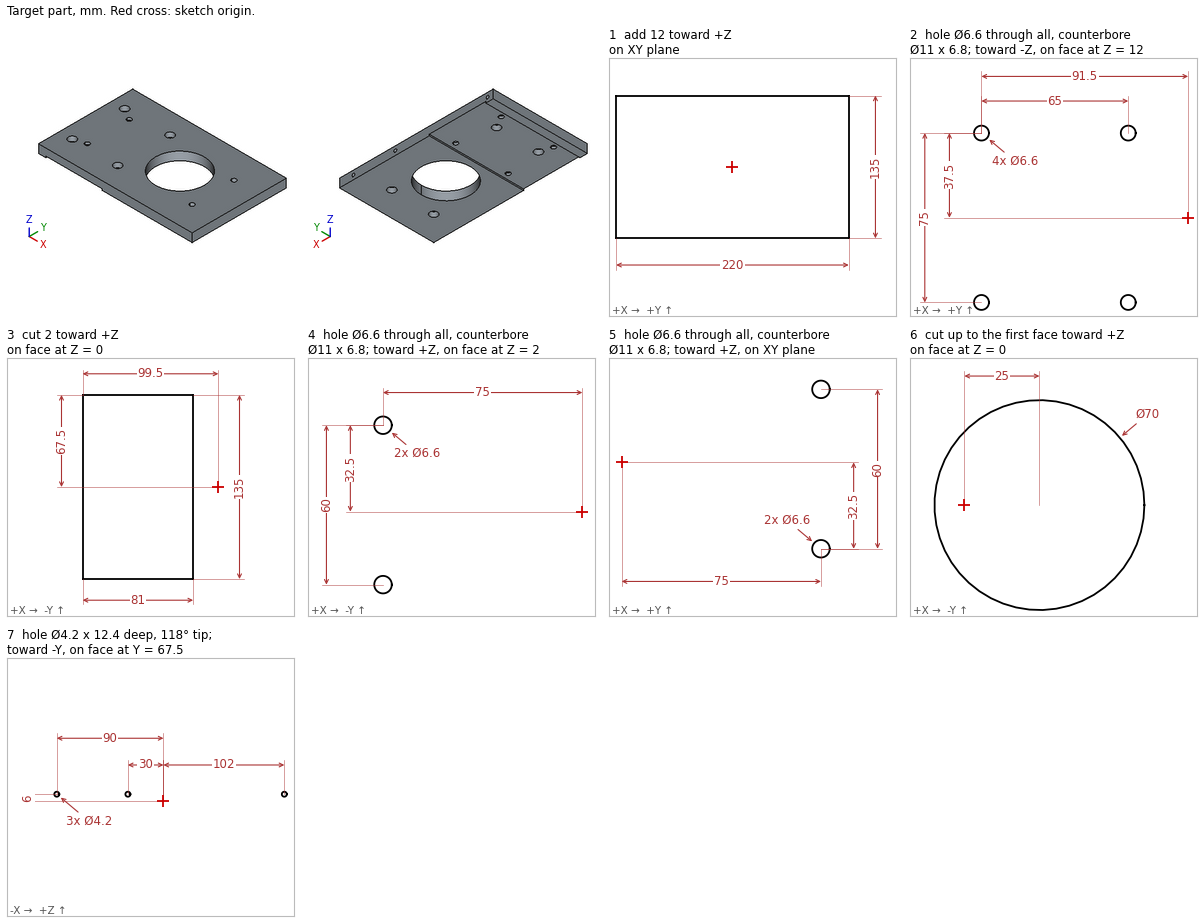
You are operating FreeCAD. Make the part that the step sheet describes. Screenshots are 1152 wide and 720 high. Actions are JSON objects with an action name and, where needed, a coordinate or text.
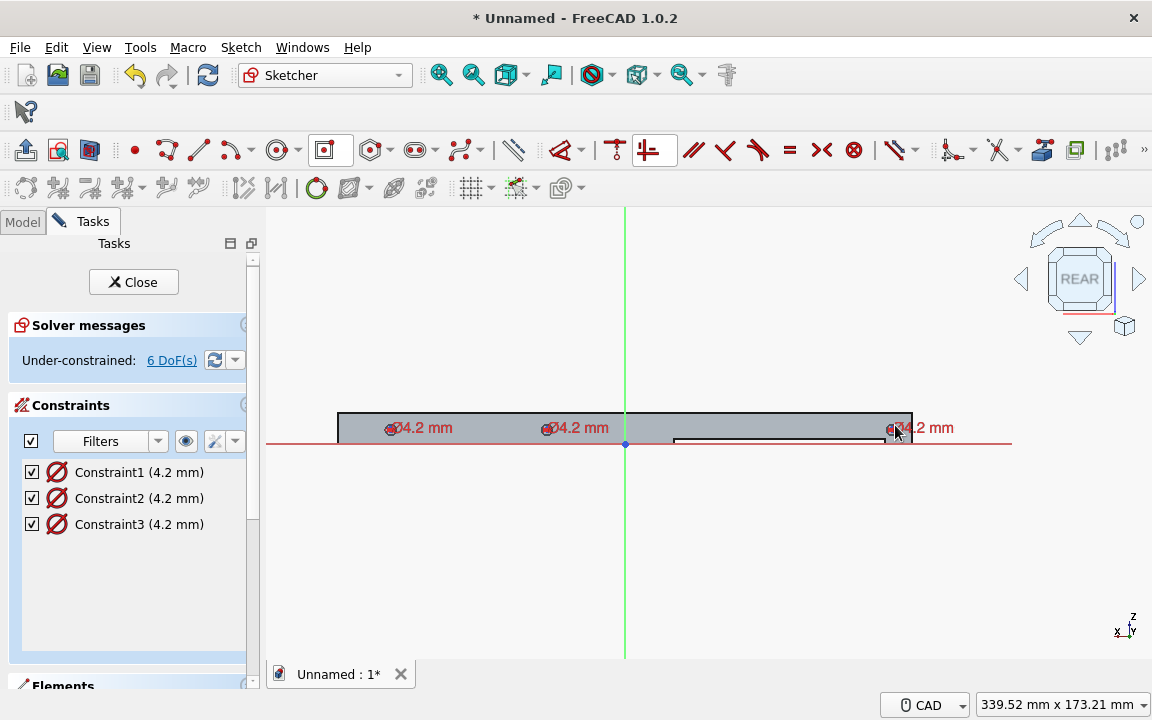
{"action": "left_click", "coordinate": [391, 430]}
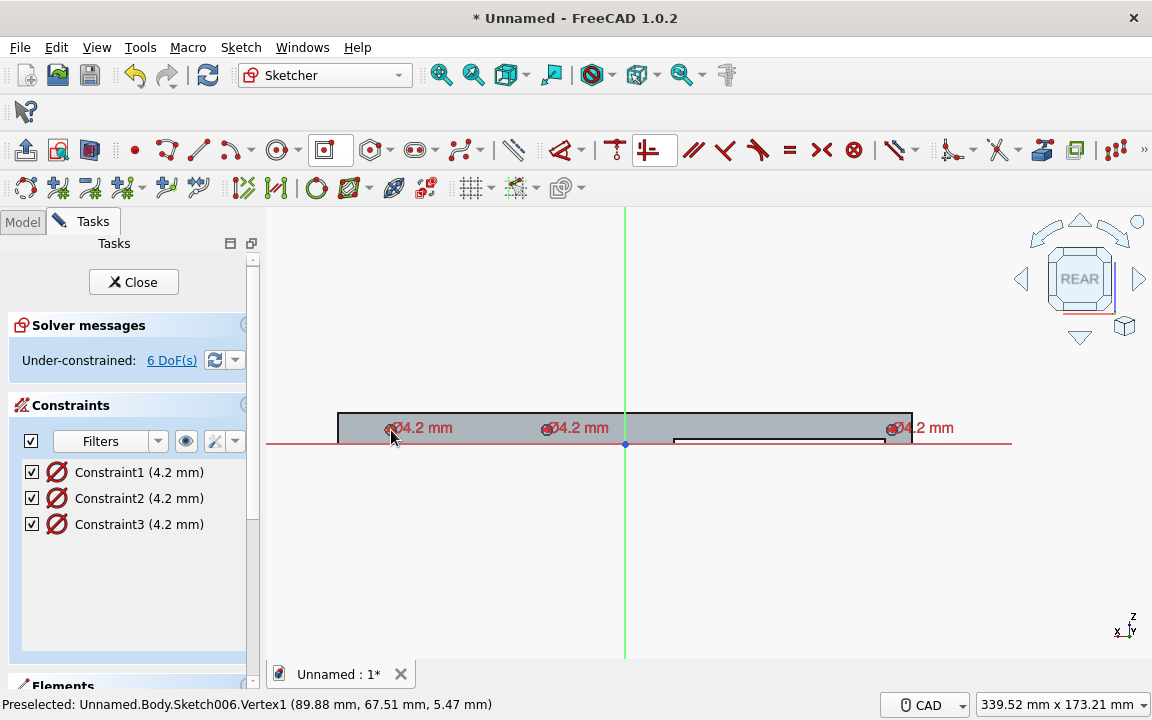
{"action": "left_click", "coordinate": [547, 430]}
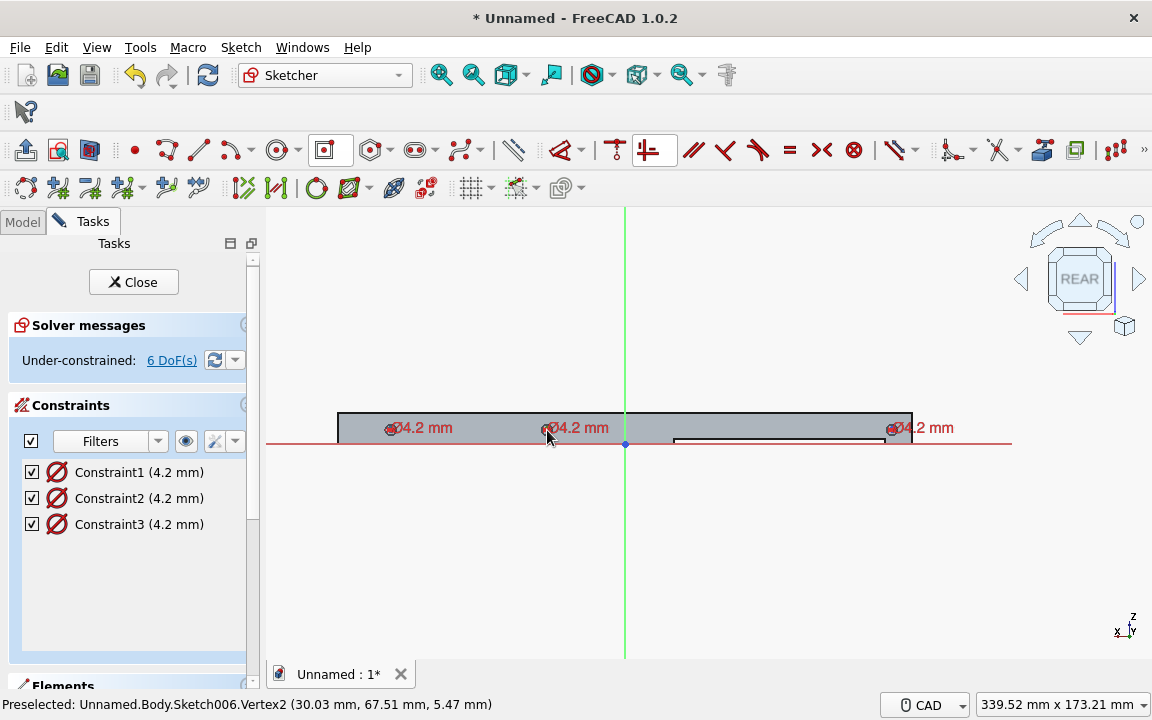
{"action": "key", "text": "h"}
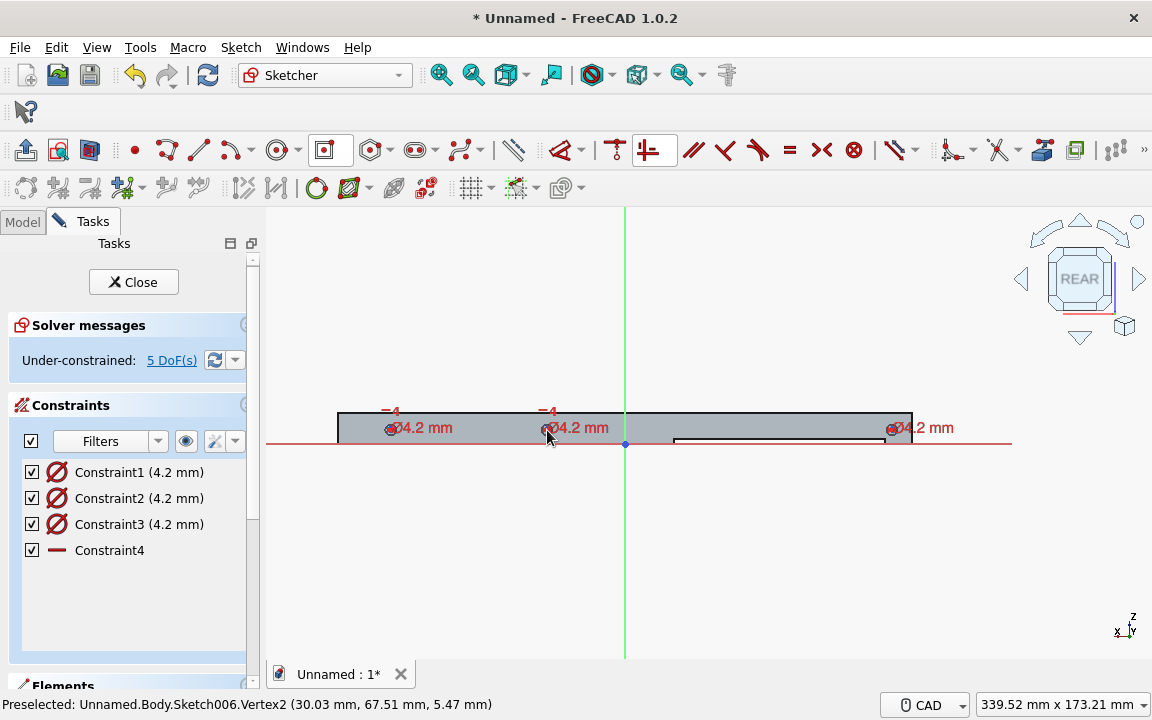
{"action": "left_click", "coordinate": [547, 430]}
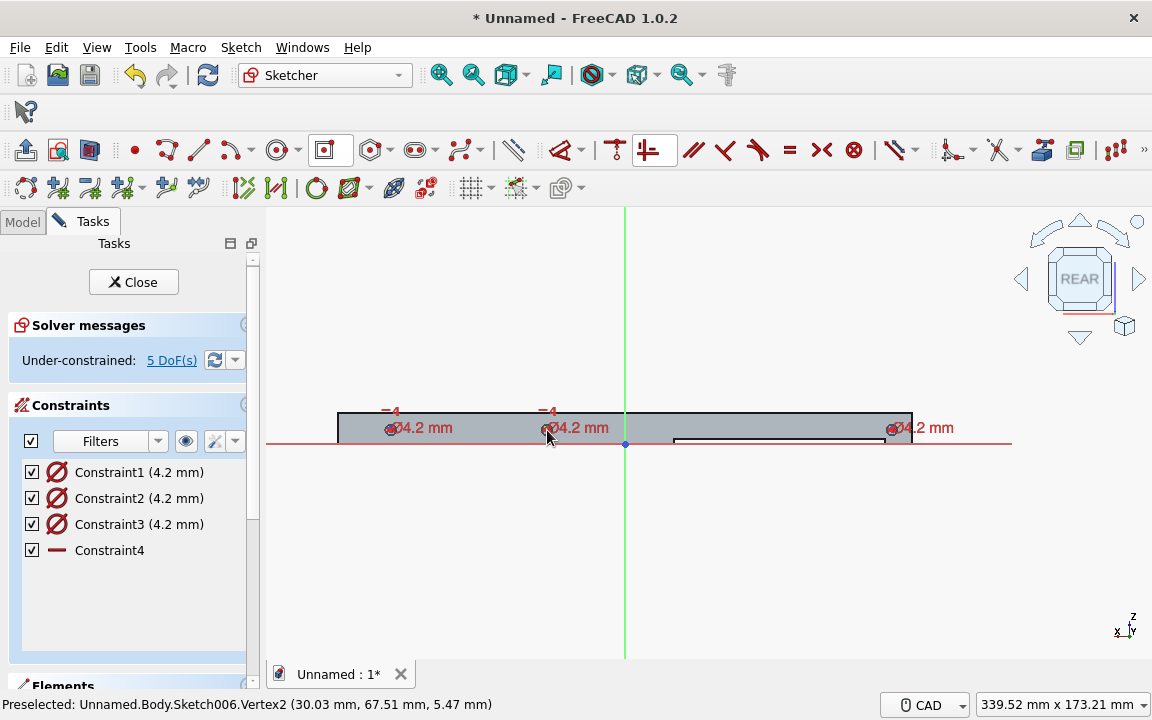
{"action": "left_click", "coordinate": [892, 430]}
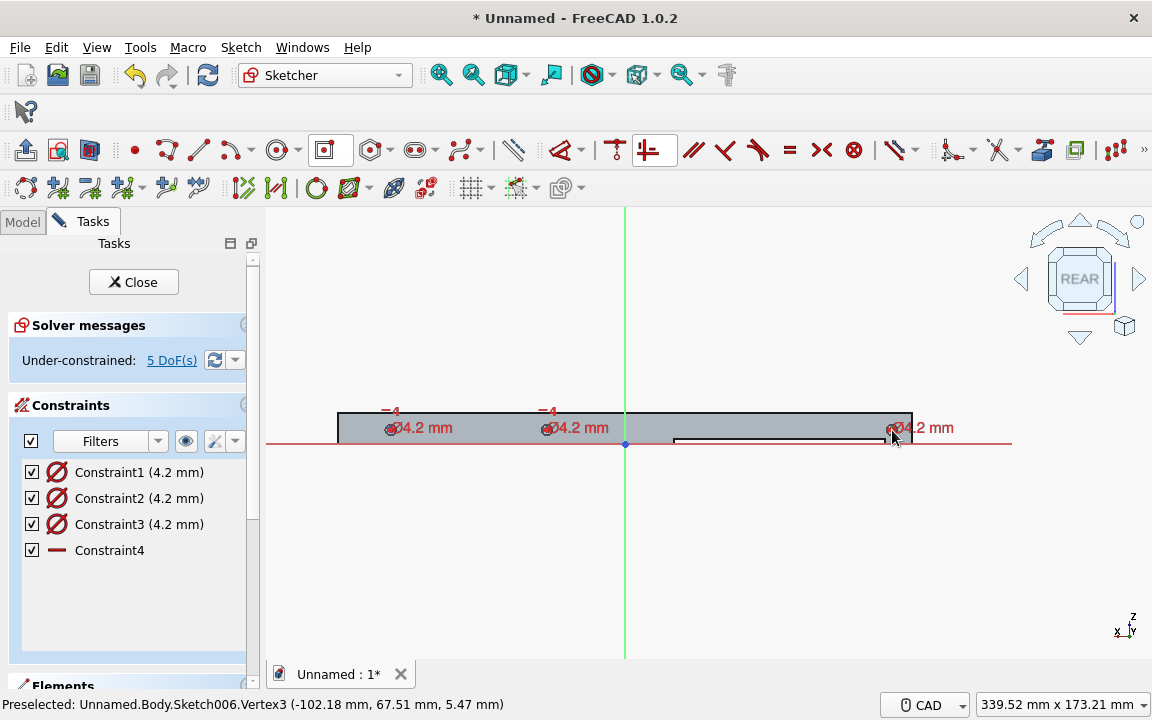
{"action": "key", "text": "h"}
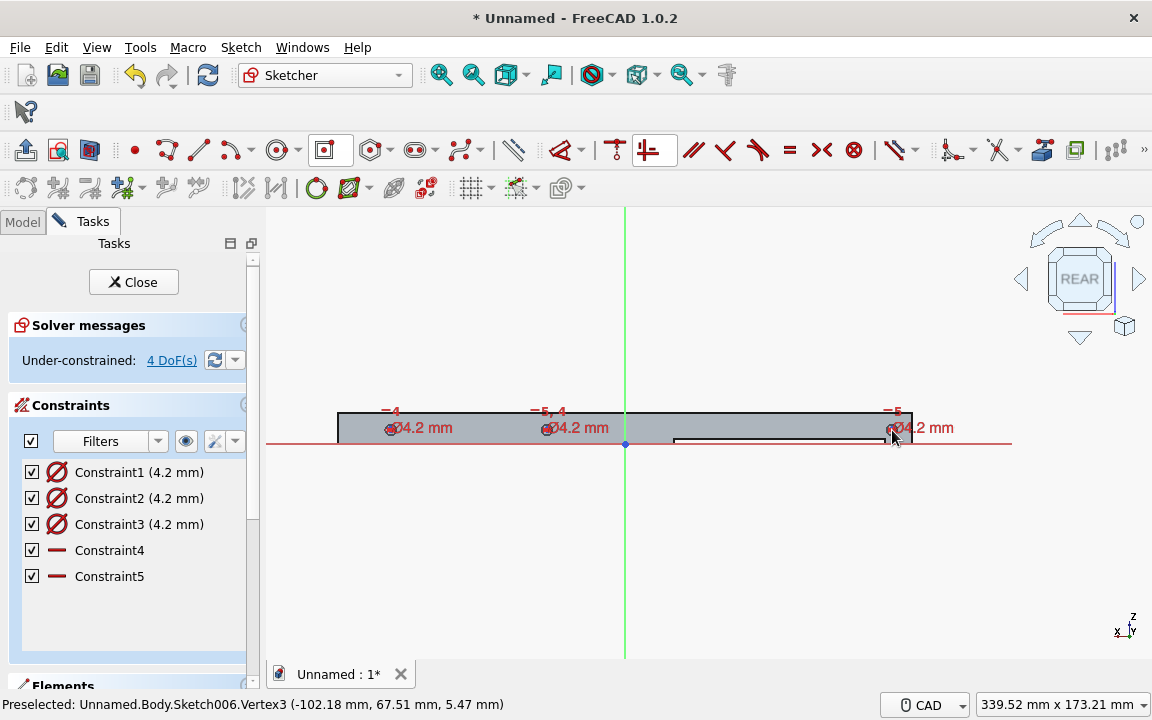
{"action": "key", "text": "d"}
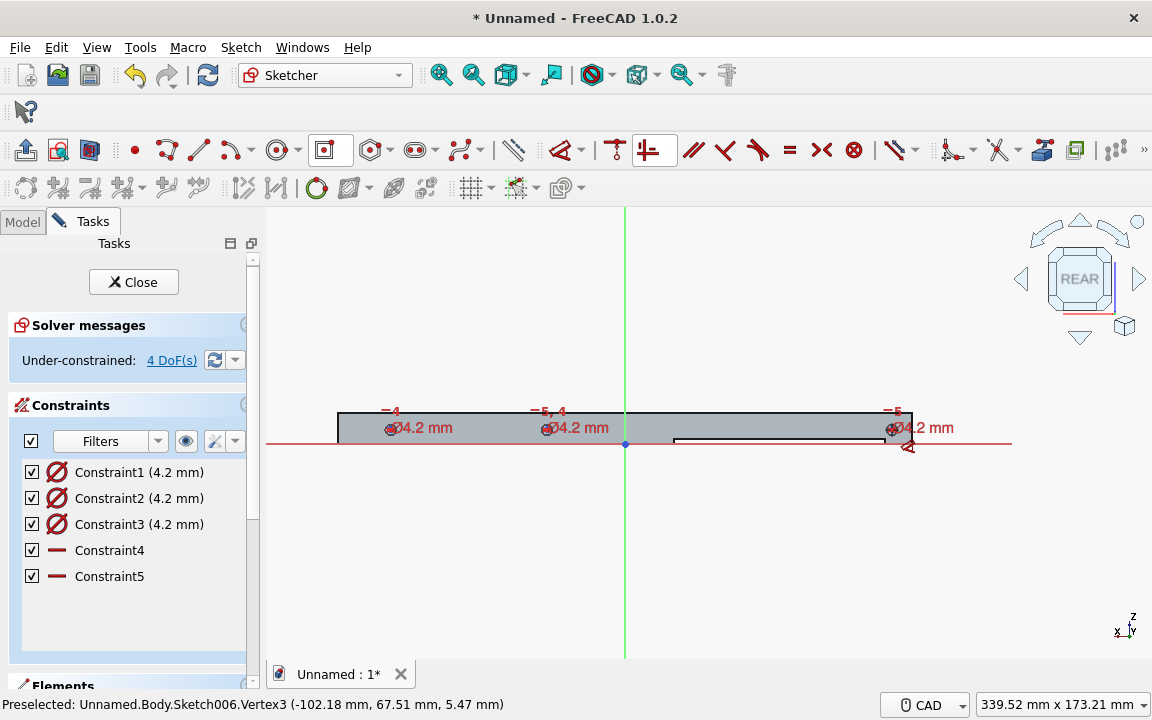
{"action": "scroll", "coordinate": [391, 430], "scroll_direction": "up", "scroll_amount": 5}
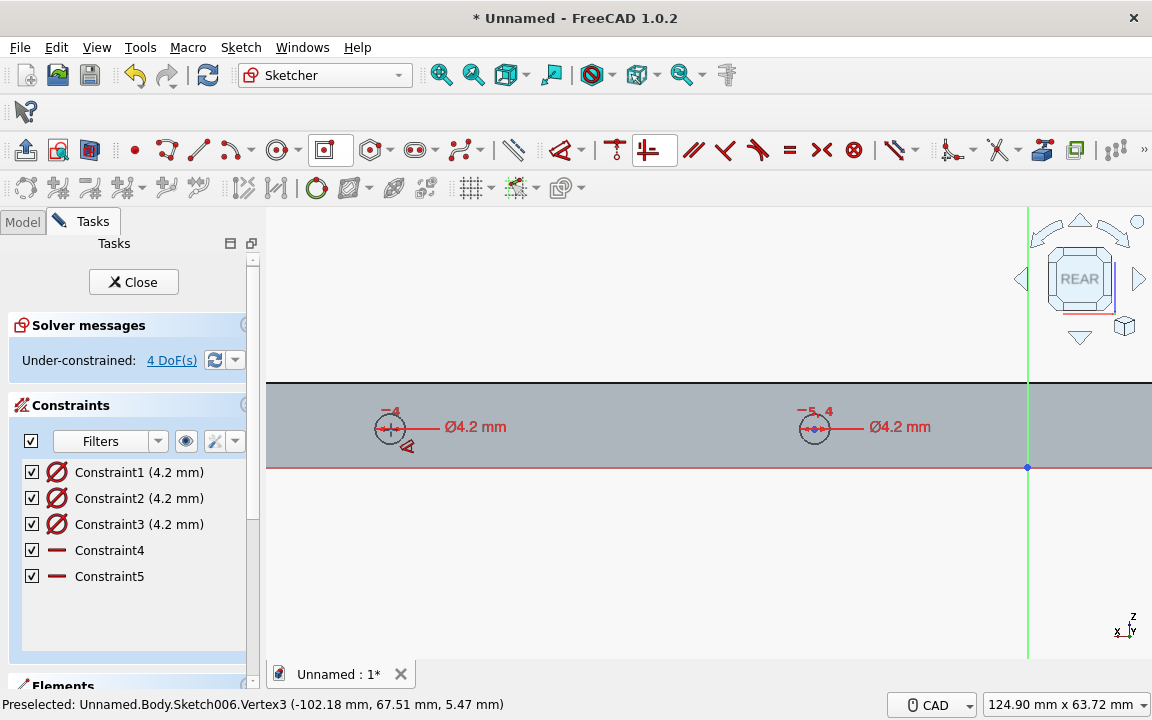
{"action": "left_click", "coordinate": [390, 429]}
{"action": "left_click", "coordinate": [356, 449]}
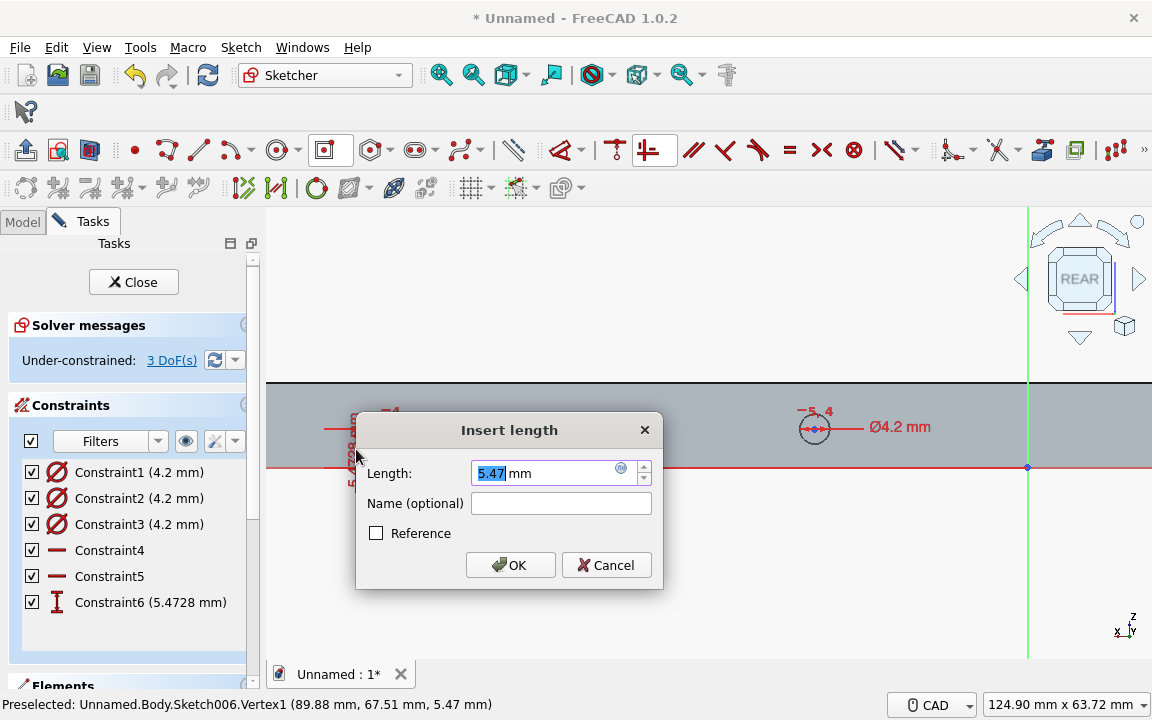
{"action": "type", "text": "6"}
{"action": "key", "text": "Return"}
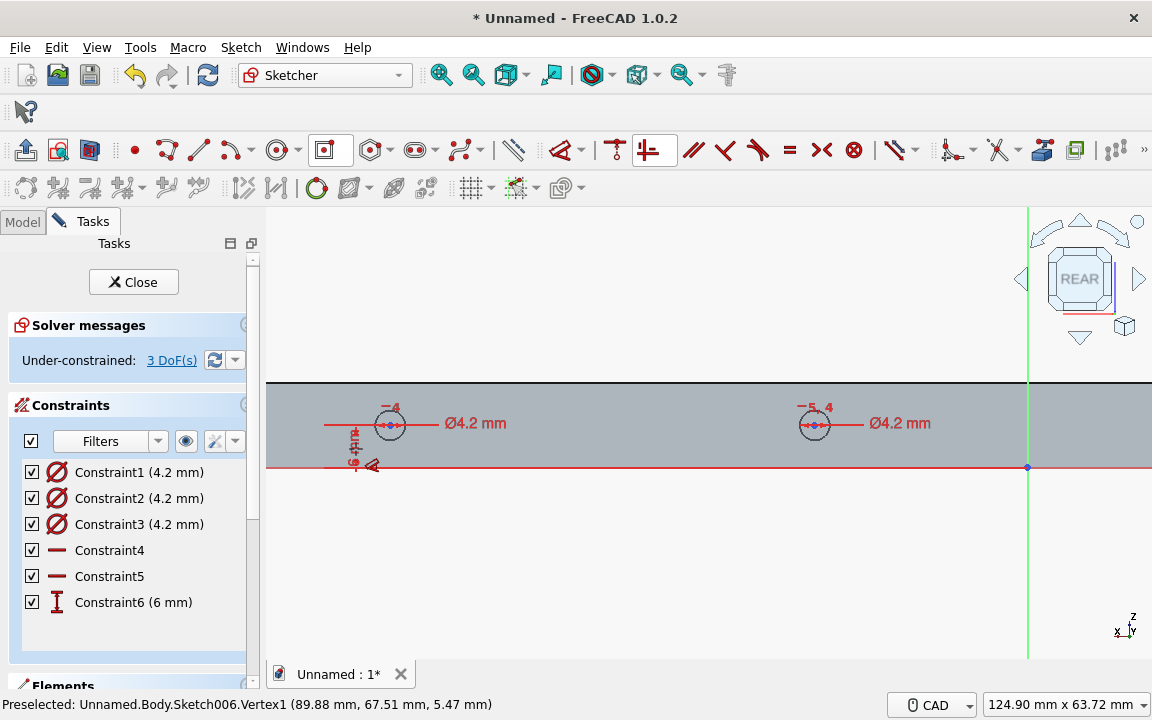
{"action": "left_click", "coordinate": [390, 425]}
{"action": "left_click", "coordinate": [689, 502]}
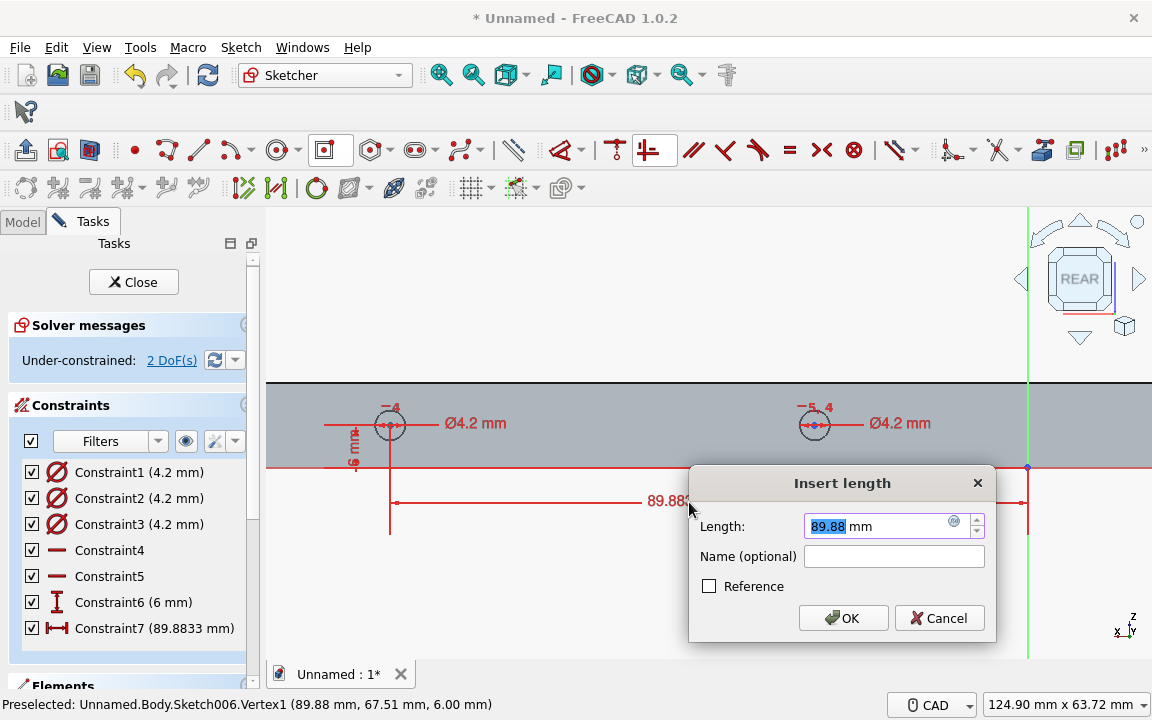
{"action": "type", "text": "90"}
{"action": "key", "text": "Return"}